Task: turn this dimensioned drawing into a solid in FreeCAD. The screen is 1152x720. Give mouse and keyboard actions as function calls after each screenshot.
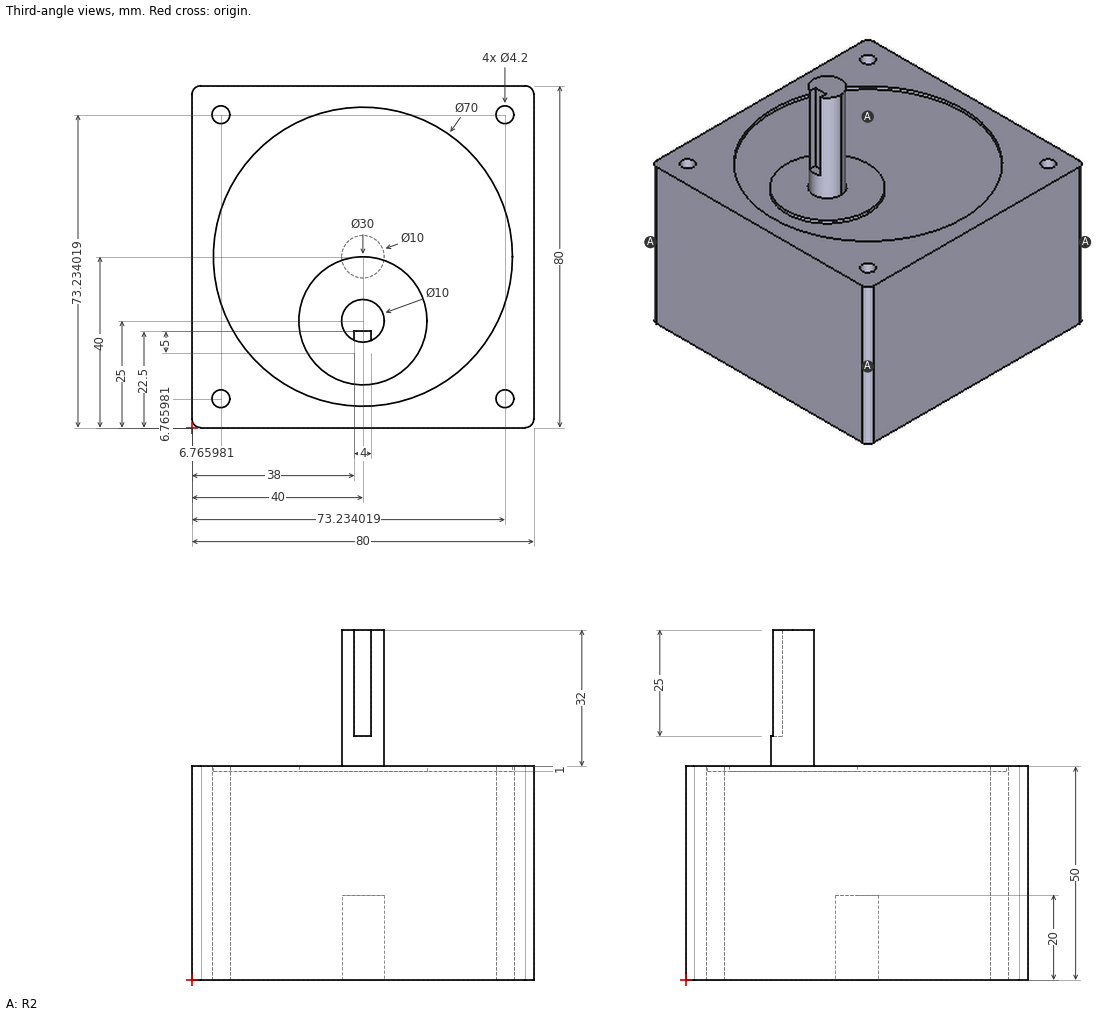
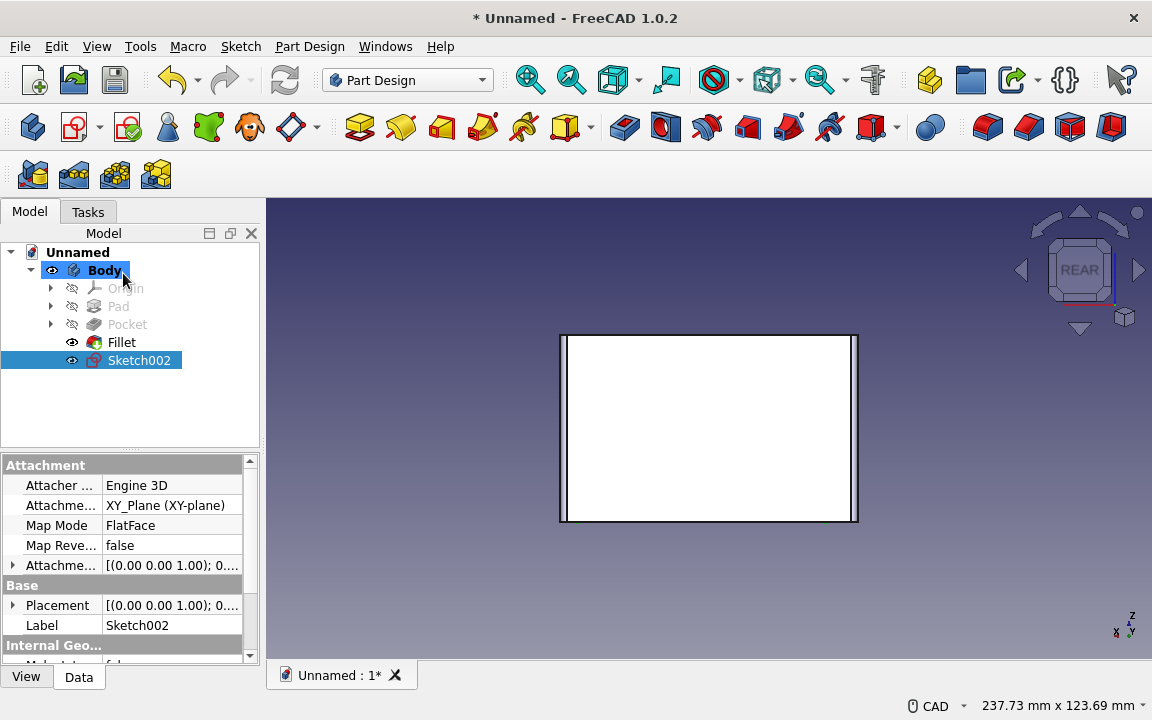
click(625, 128)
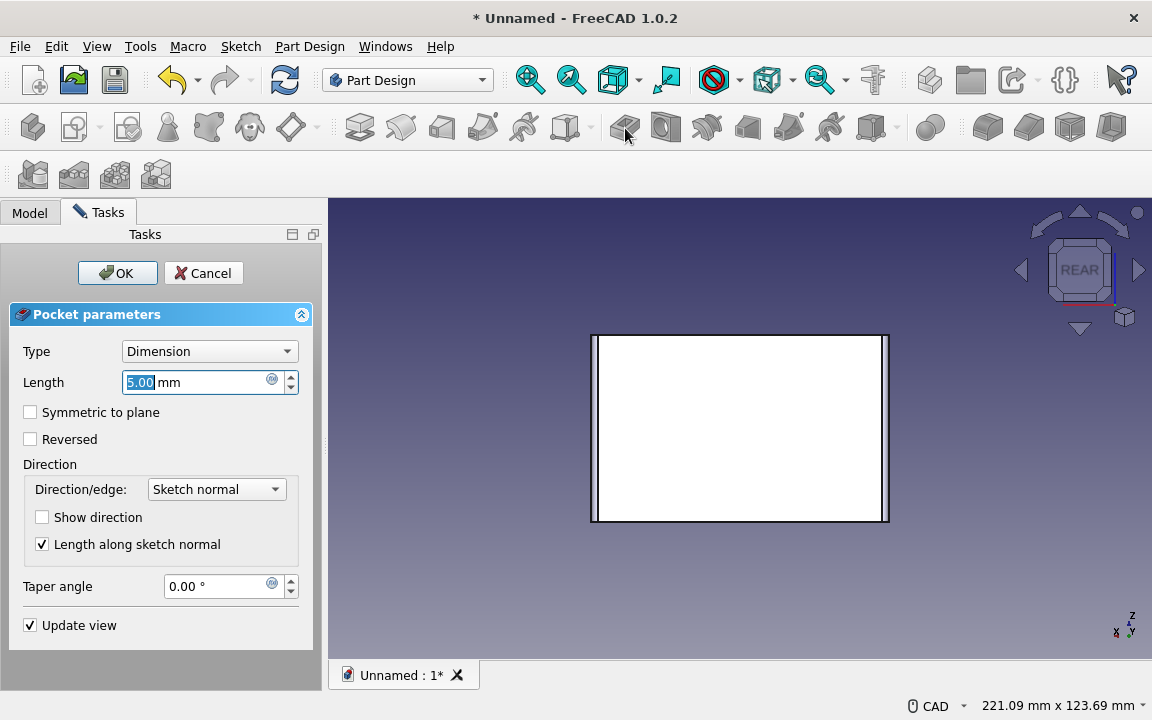
click(210, 352)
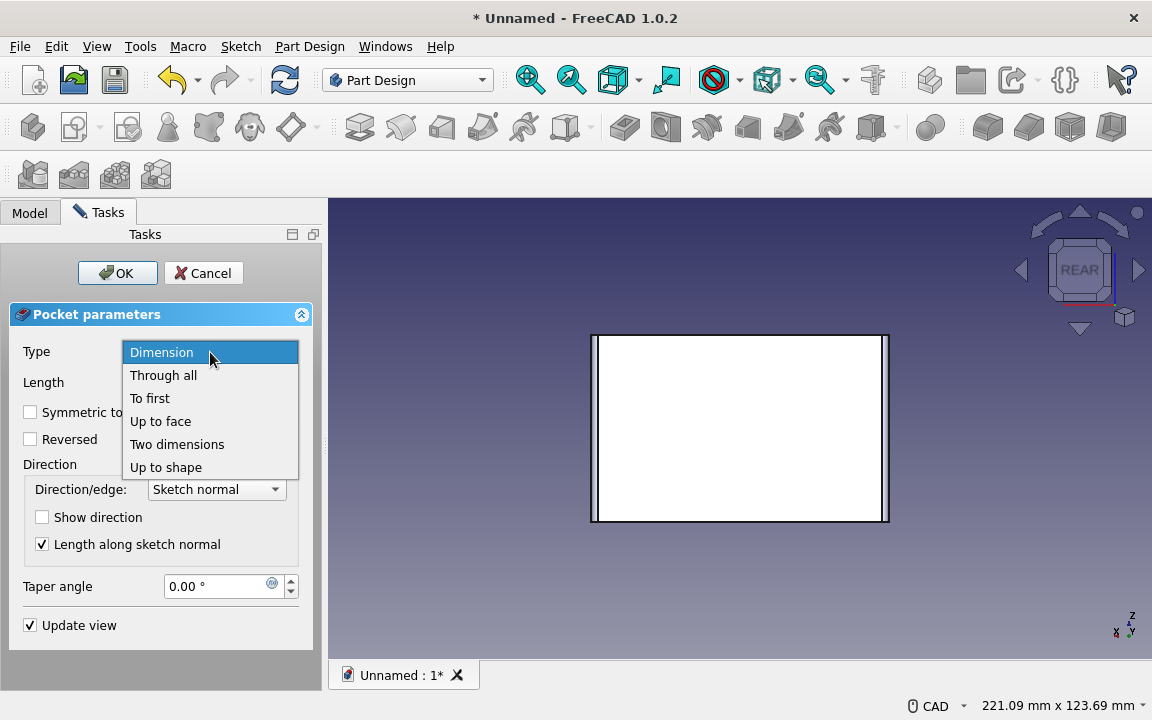
click(208, 376)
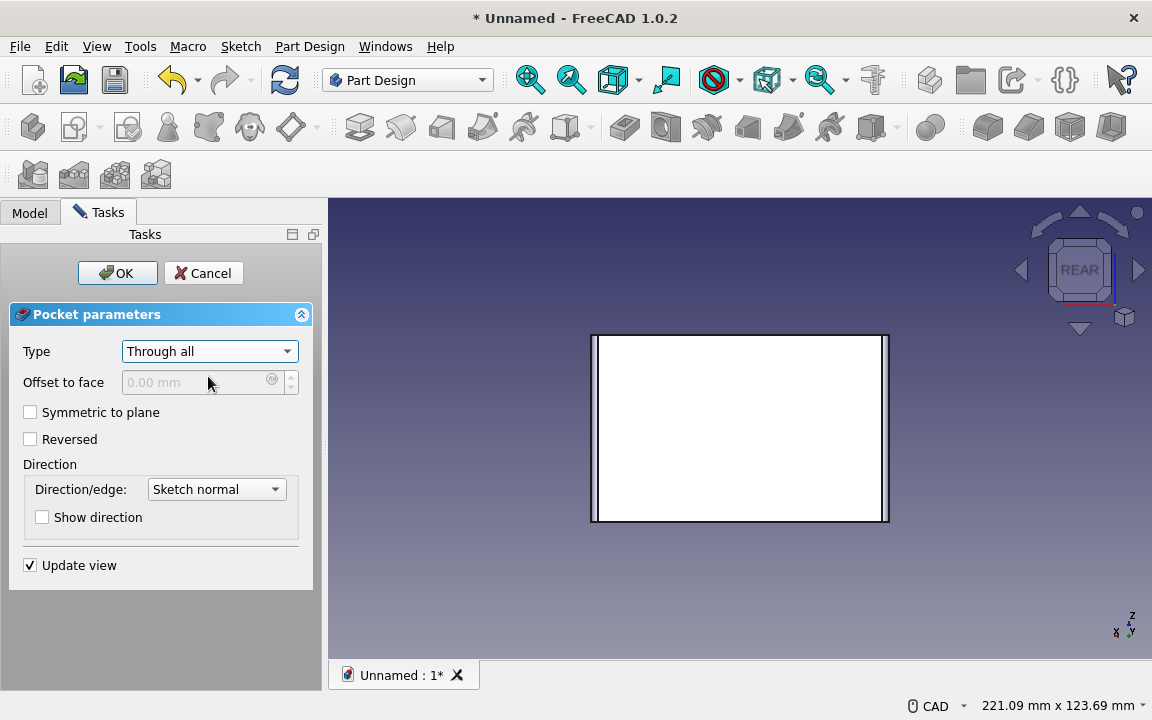
click(31, 439)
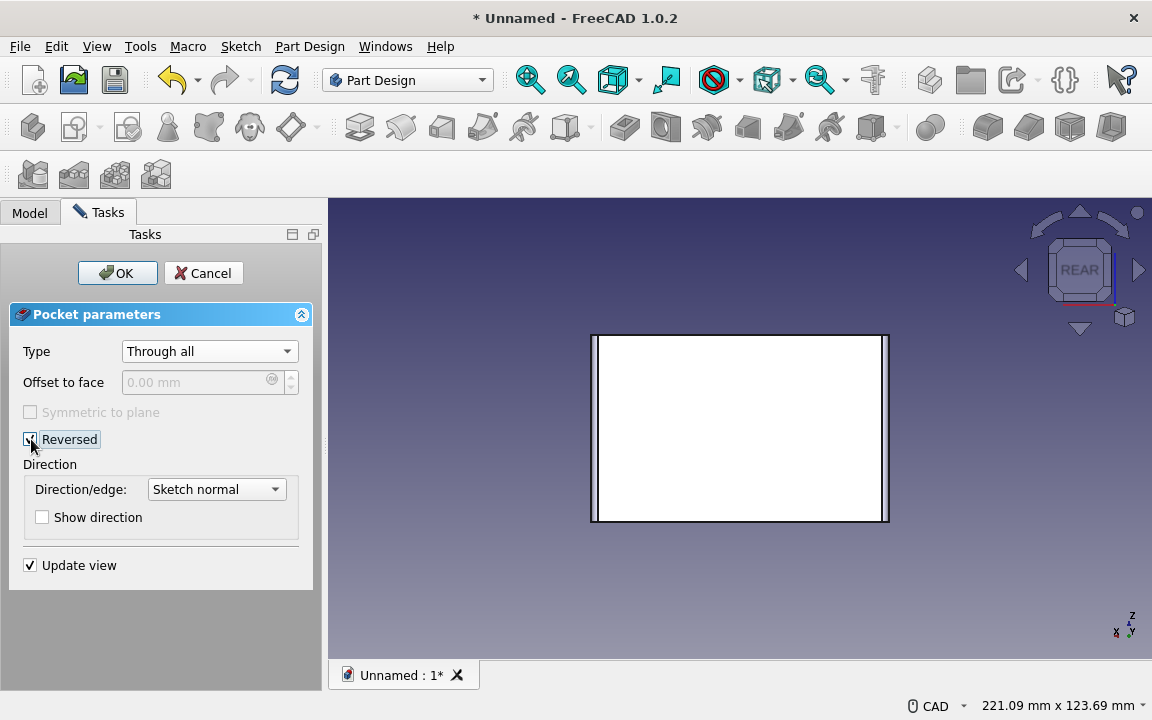
click(118, 273)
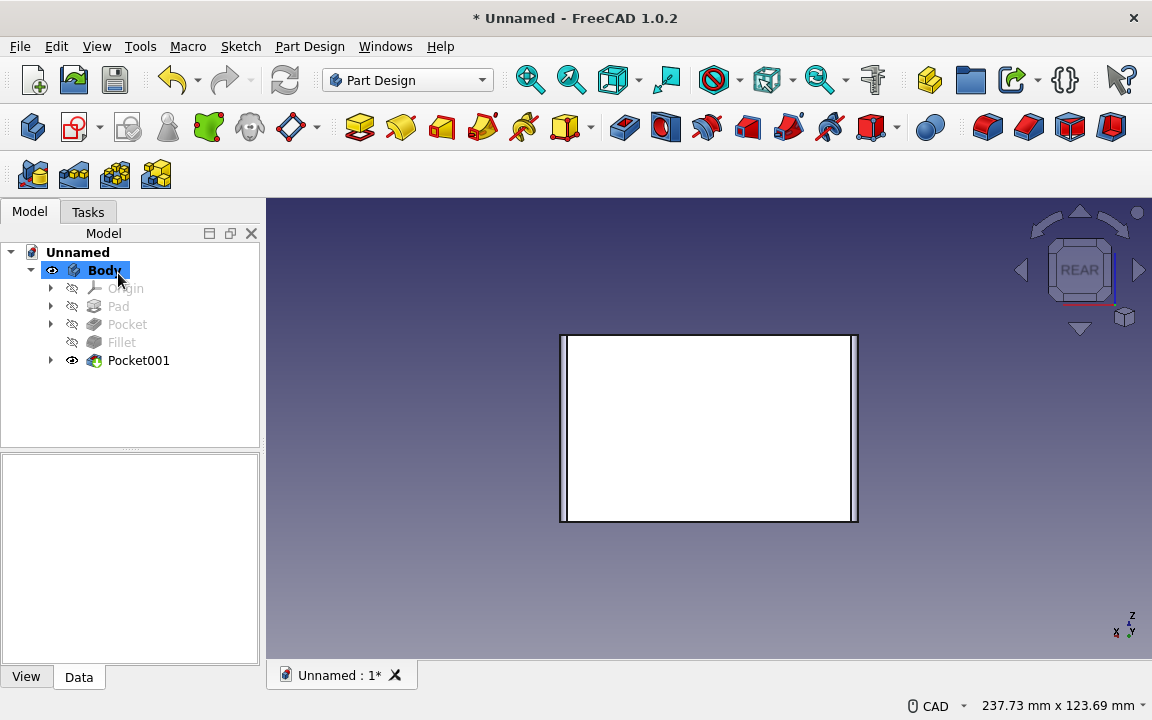
click(531, 80)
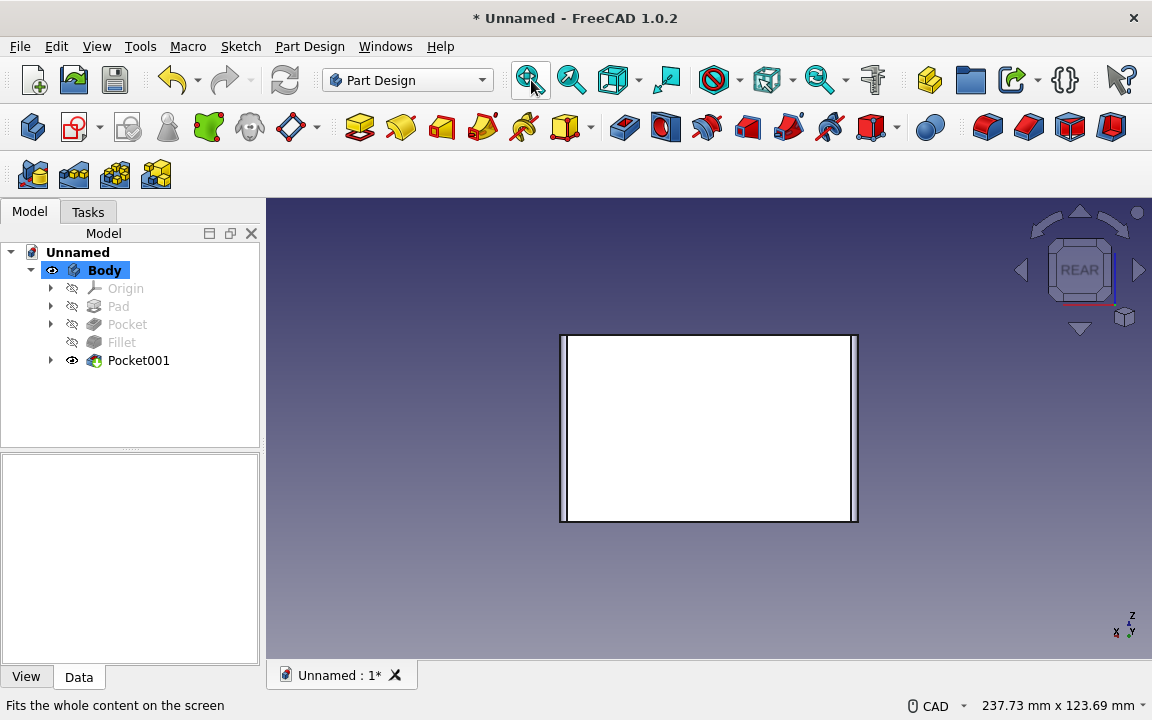
click(74, 128)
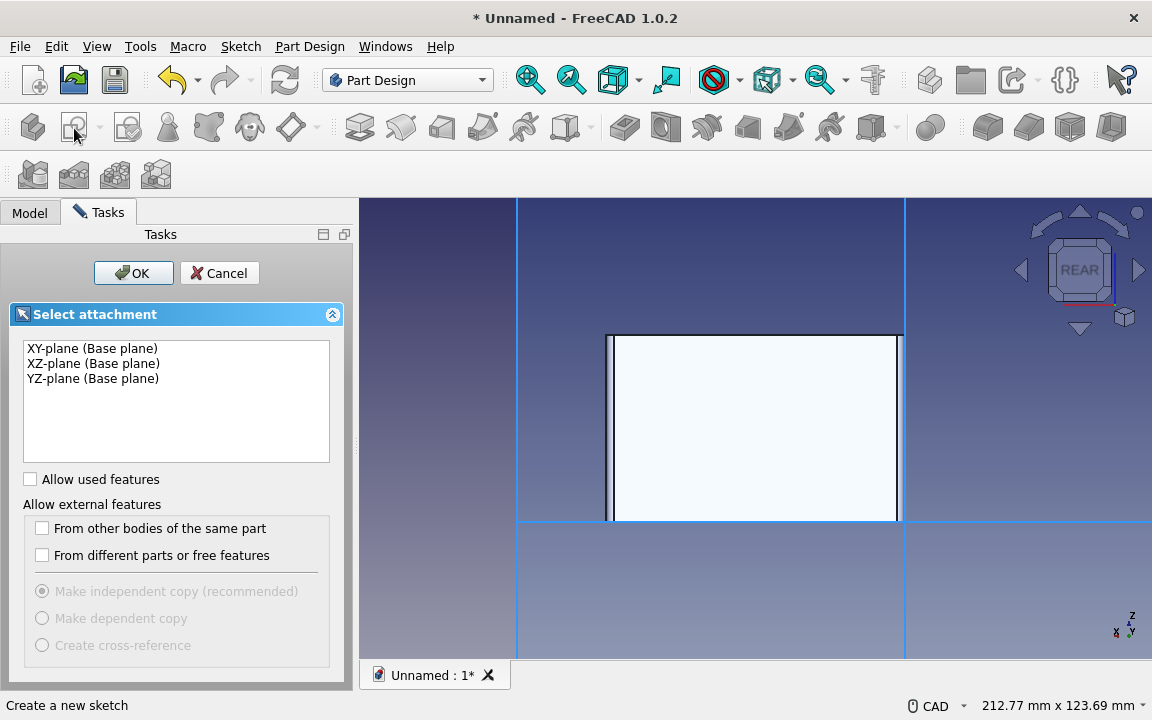
click(84, 348)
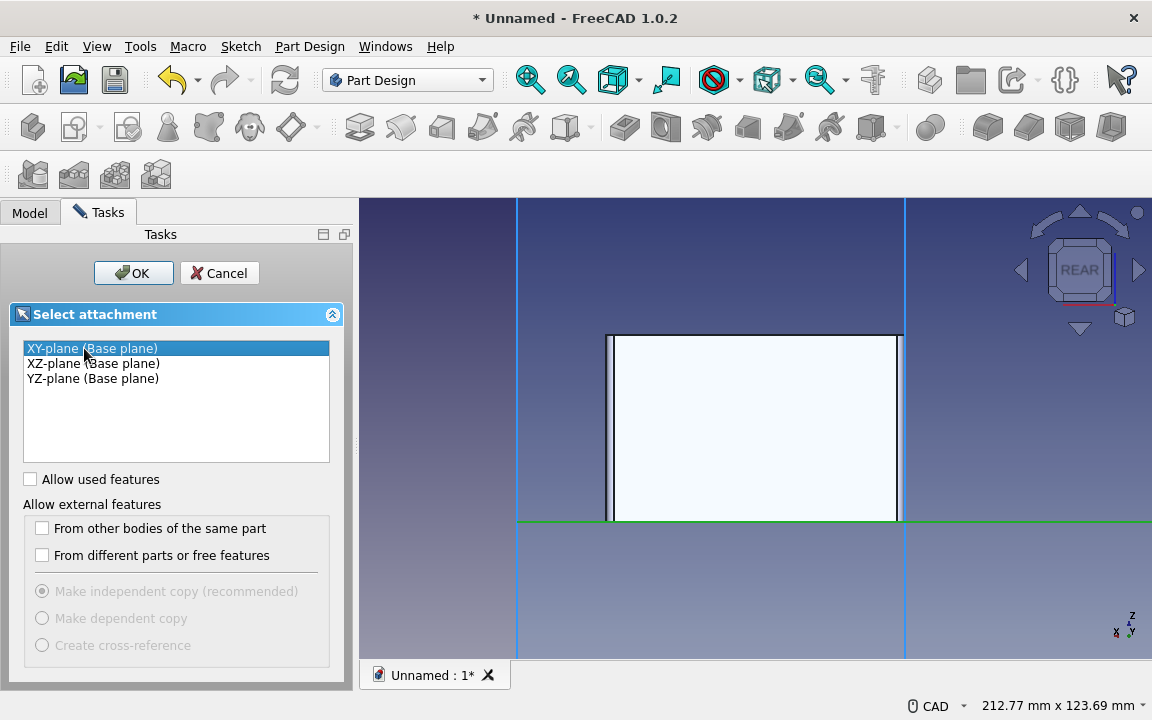
click(134, 273)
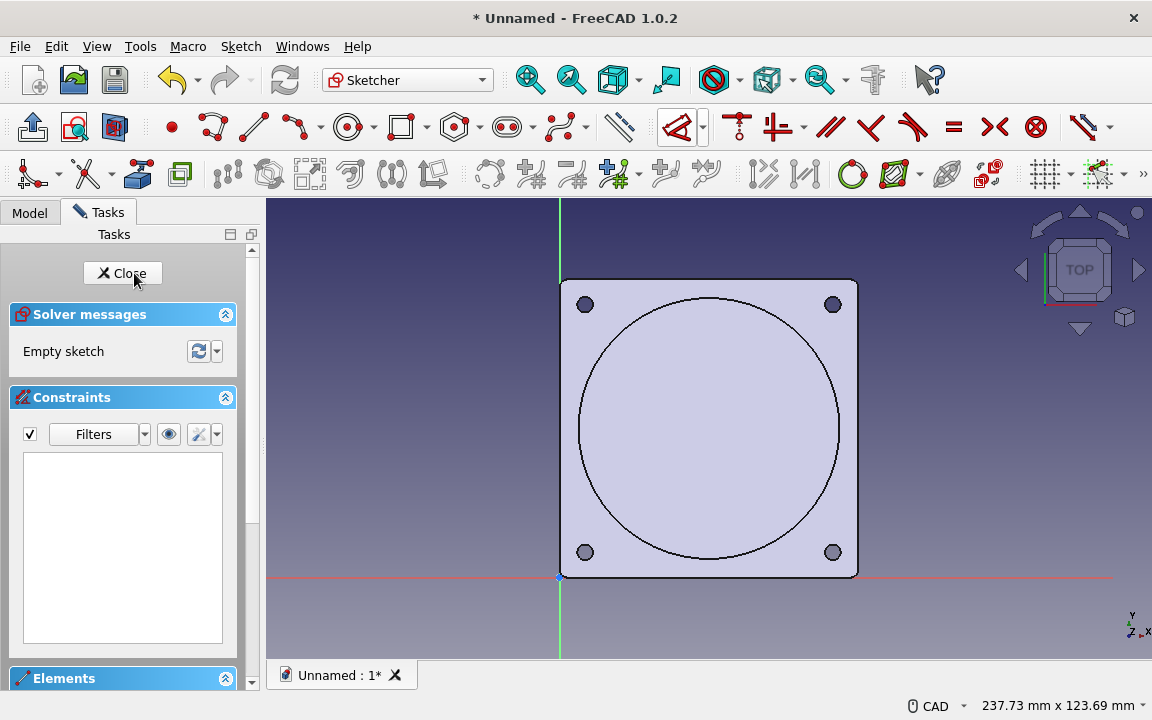
click(115, 128)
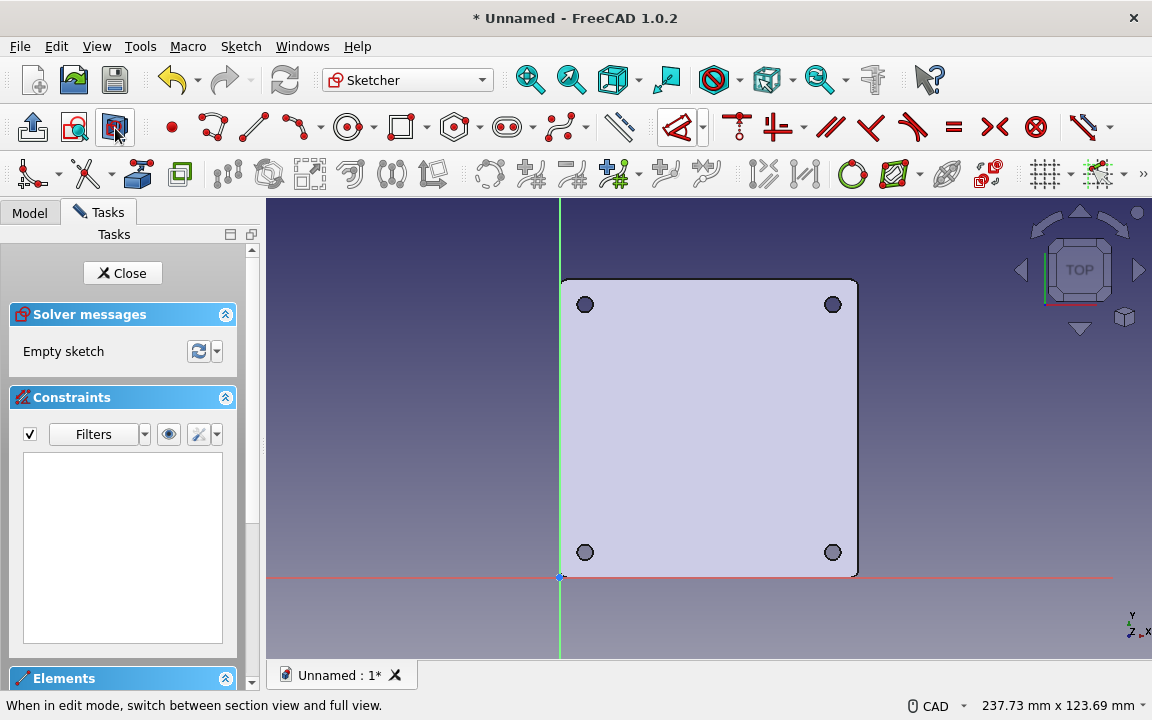
scroll(720, 428, up, 10)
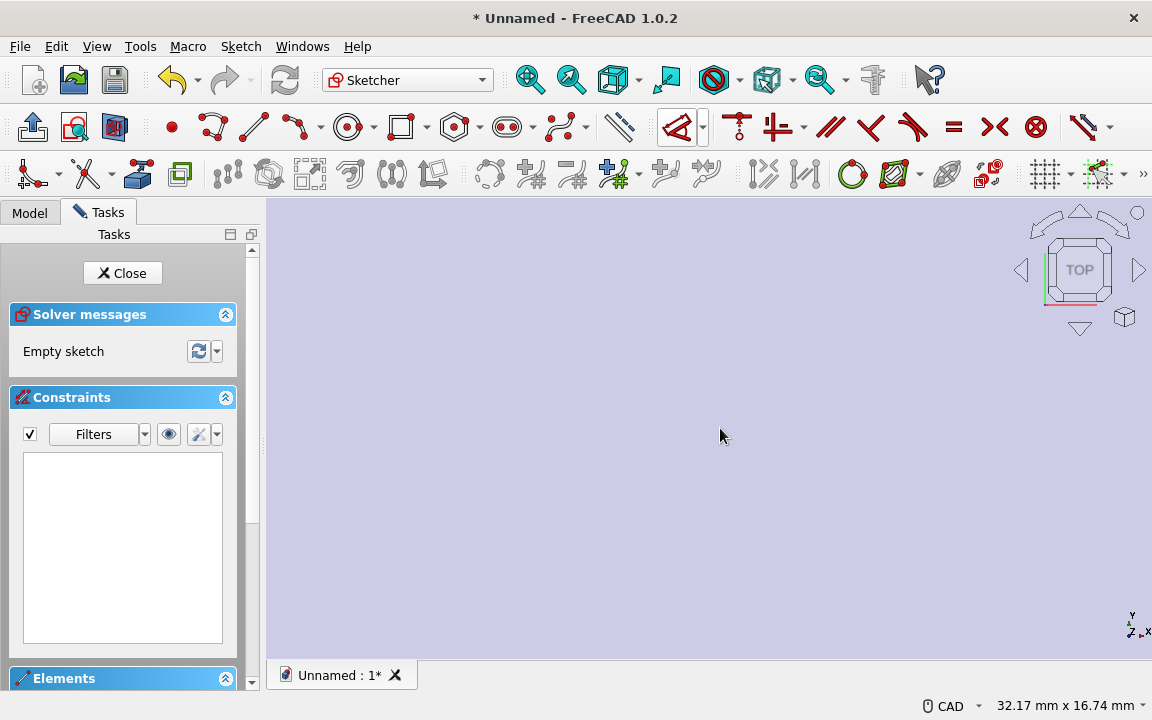
click(348, 128)